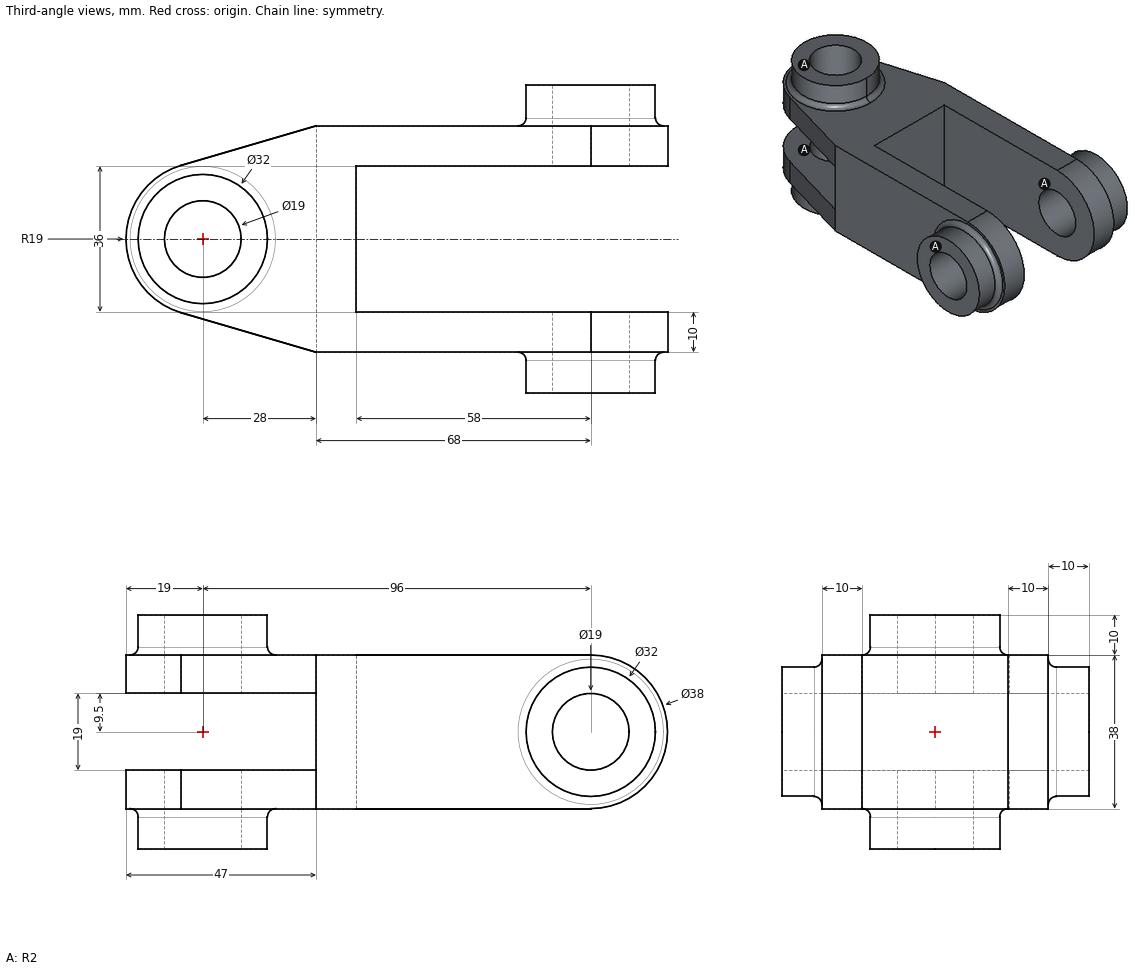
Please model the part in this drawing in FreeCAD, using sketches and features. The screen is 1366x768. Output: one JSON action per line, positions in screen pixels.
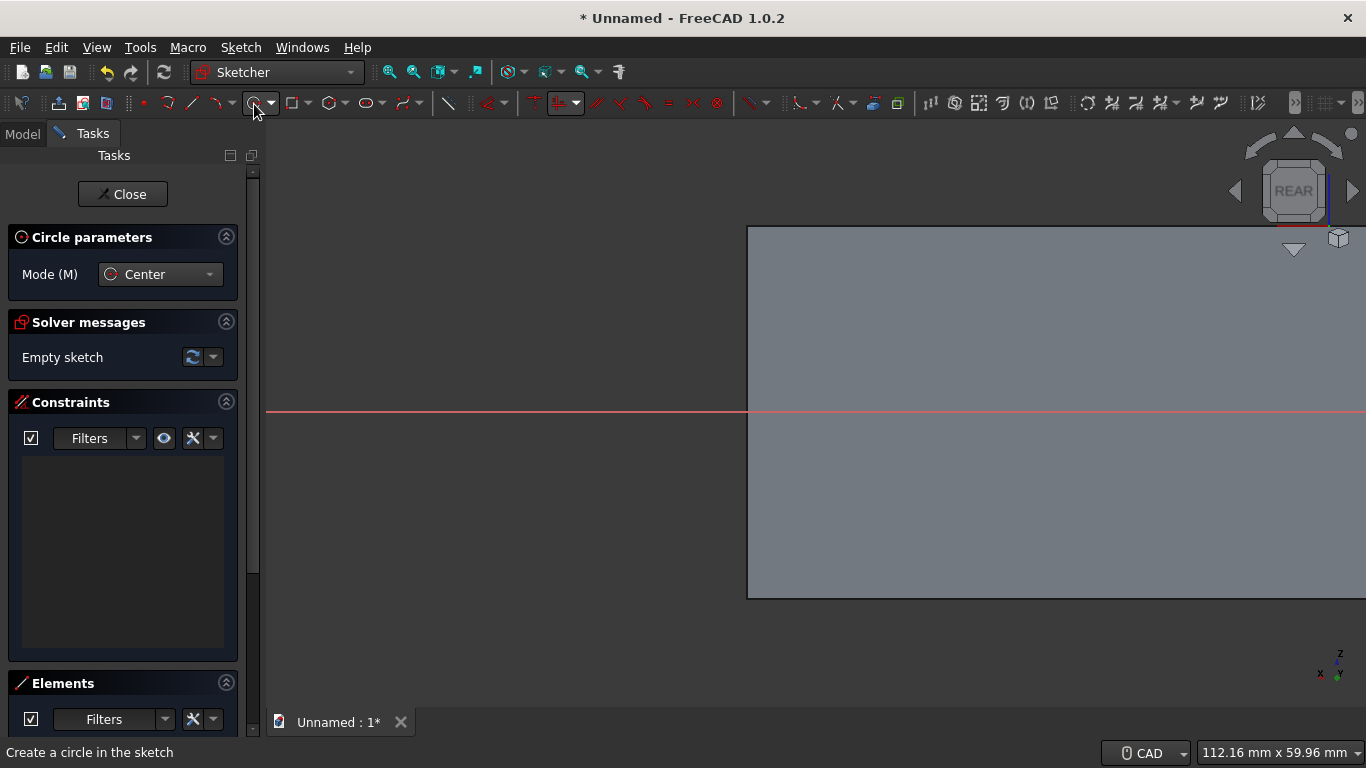
{"action": "left_click", "coordinate": [747, 412]}
{"action": "left_click", "coordinate": [879, 281]}
{"action": "key", "text": "Escape"}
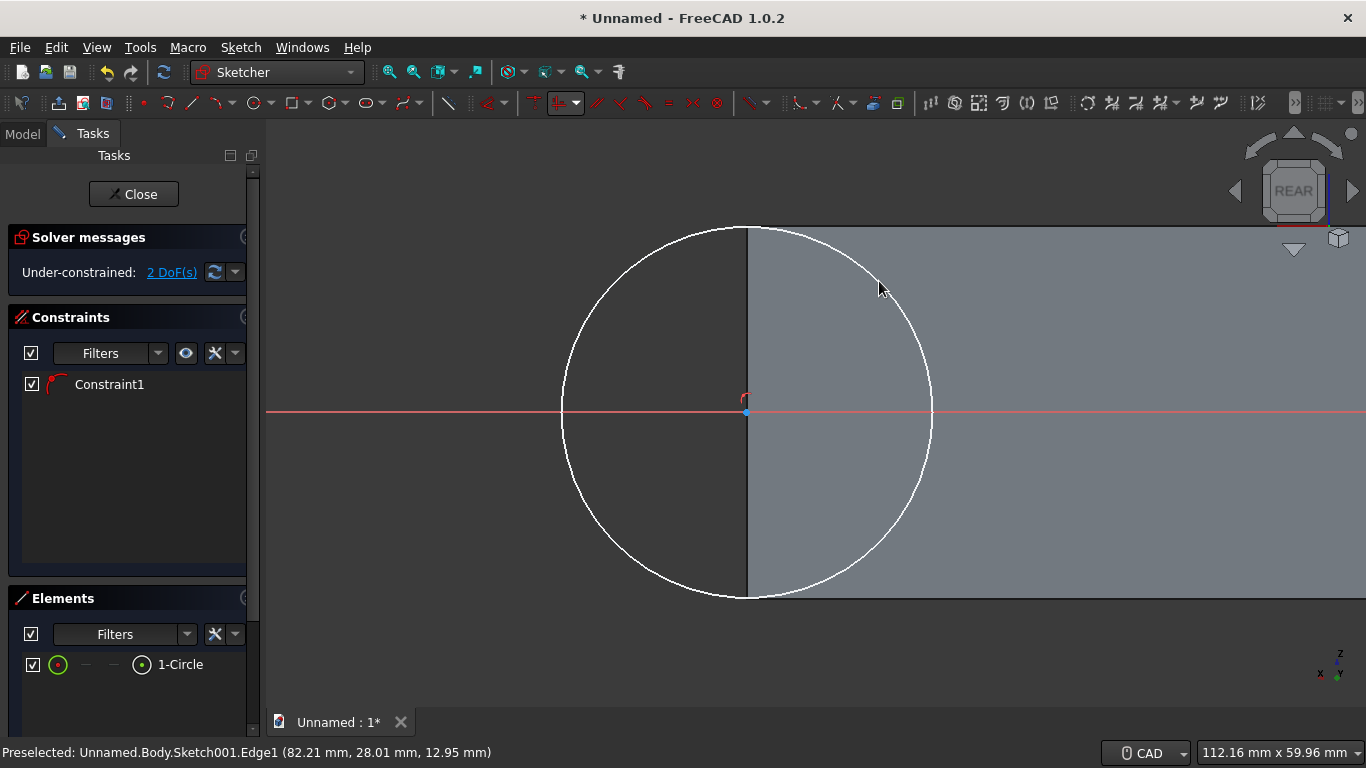
{"action": "key", "text": "d"}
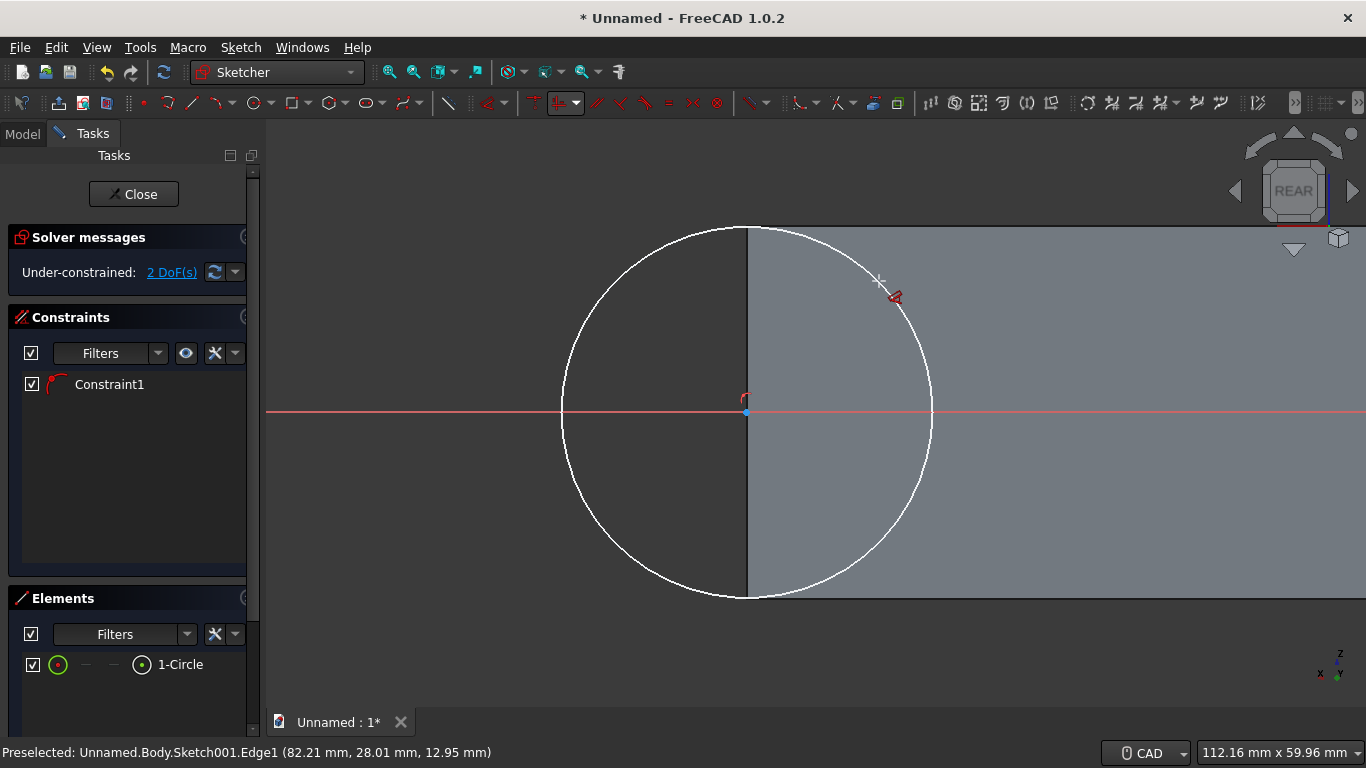
{"action": "left_click", "coordinate": [878, 281]}
{"action": "left_click", "coordinate": [901, 258]}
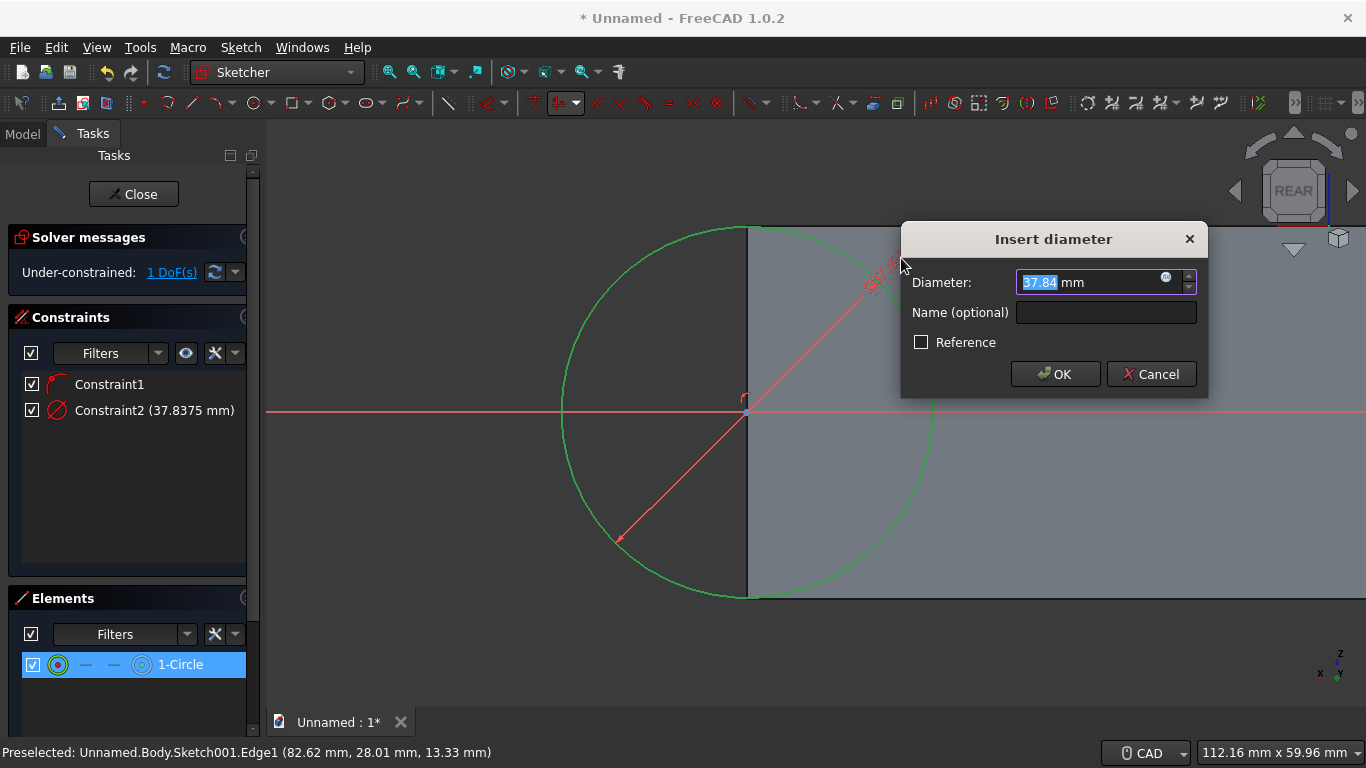
{"action": "type", "text": "38"}
{"action": "key", "text": "Return"}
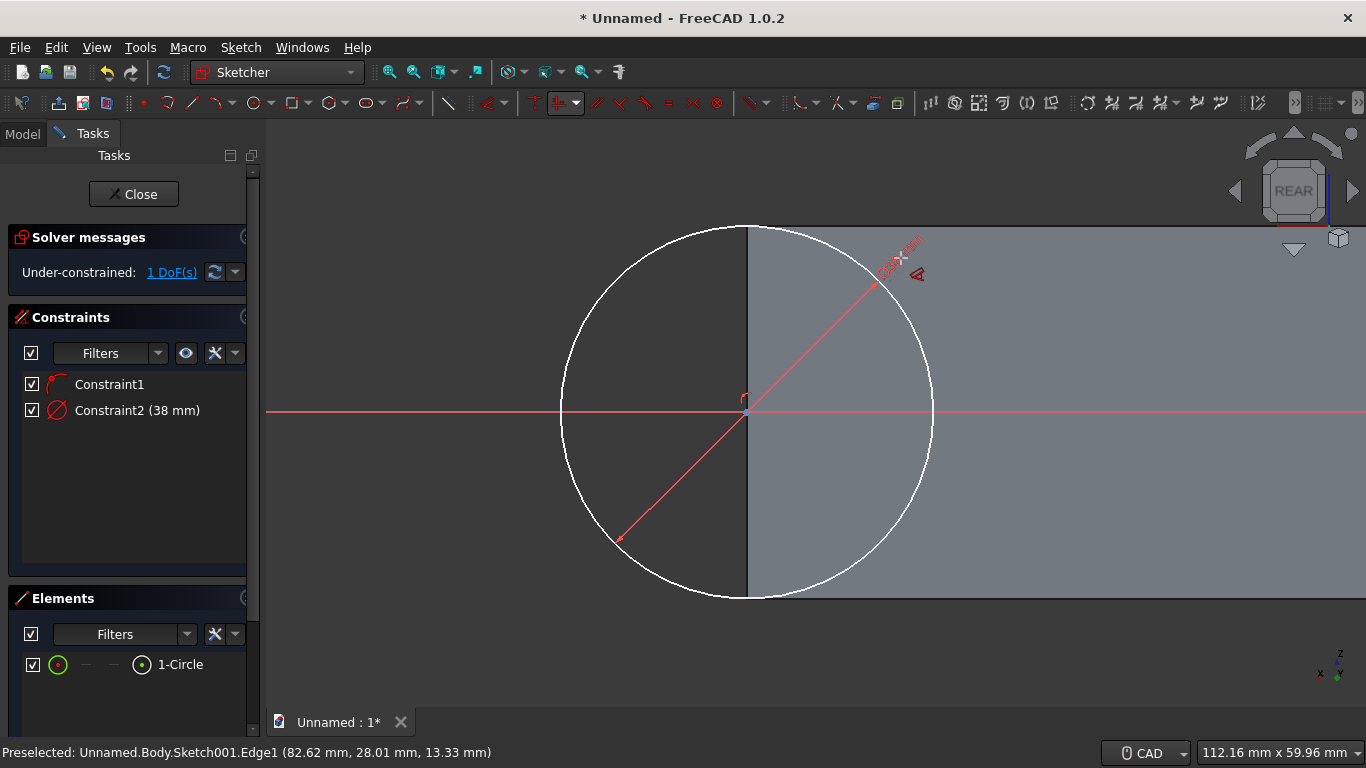
{"action": "left_click", "coordinate": [747, 412]}
{"action": "left_click", "coordinate": [974, 446]}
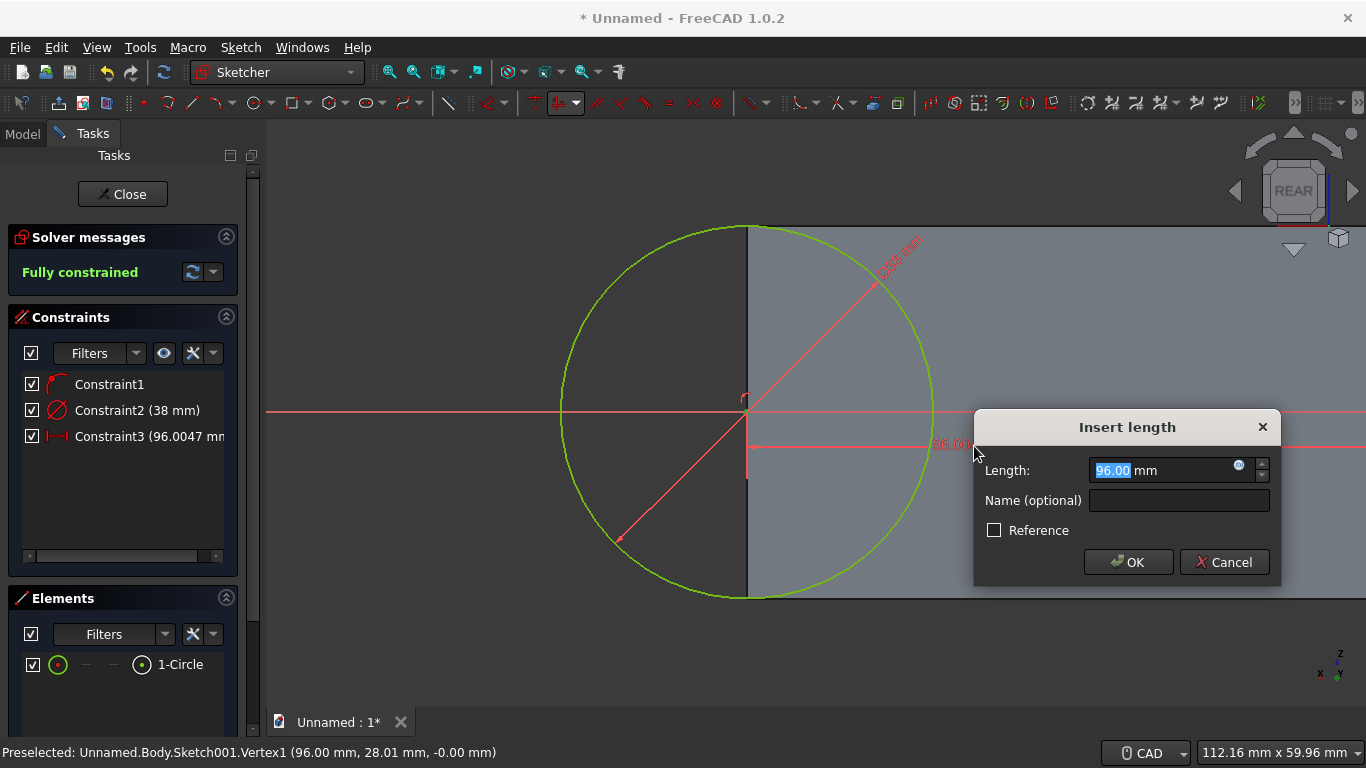
{"action": "type", "text": "96"}
{"action": "key", "text": "Return"}
{"action": "key", "text": "Escape"}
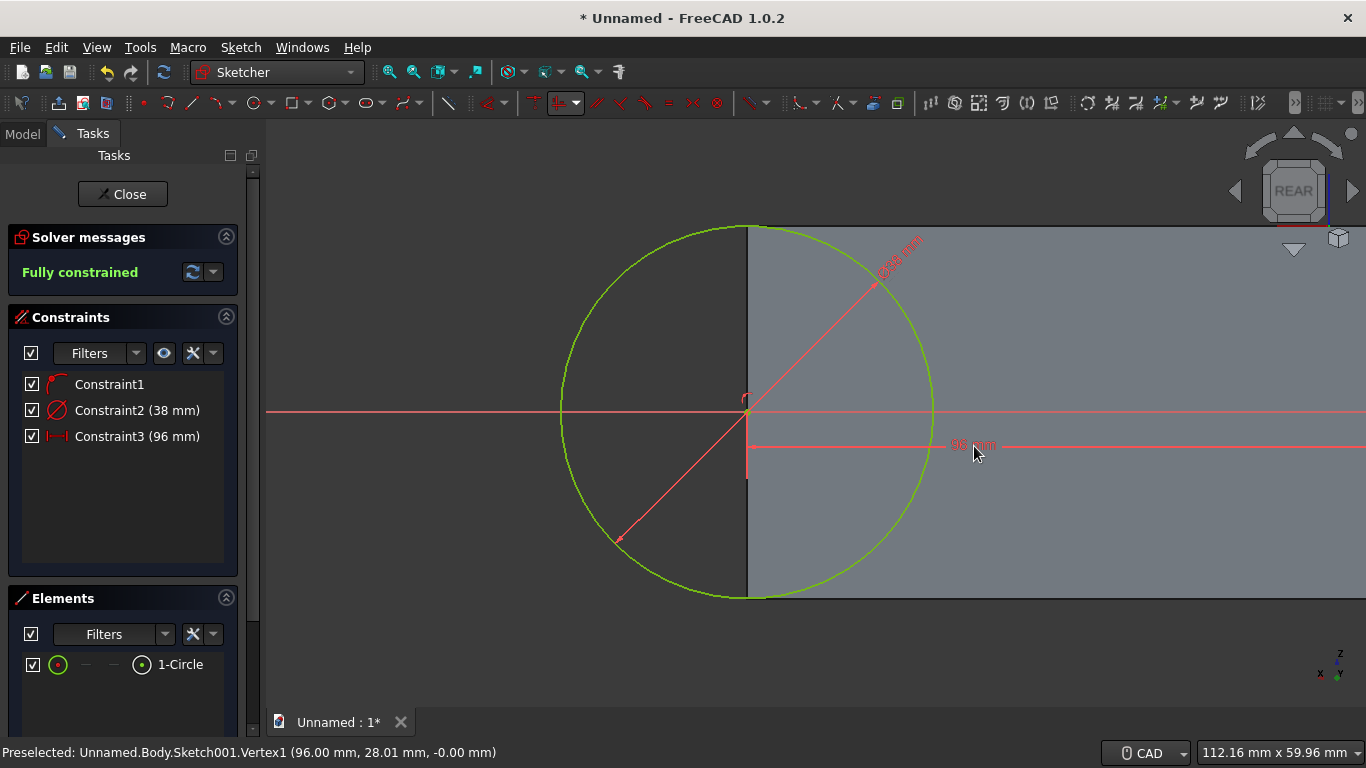
{"action": "left_click", "coordinate": [123, 194]}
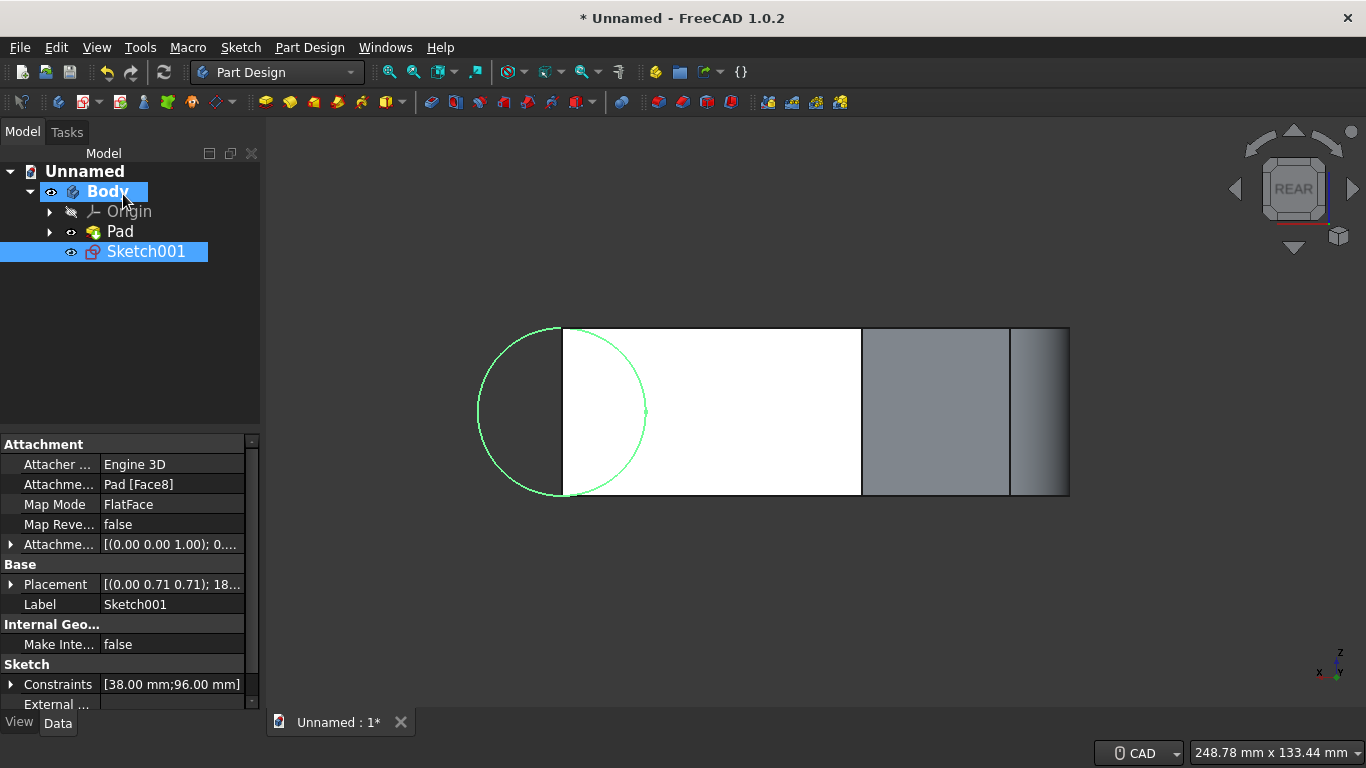
{"action": "left_click", "coordinate": [266, 102]}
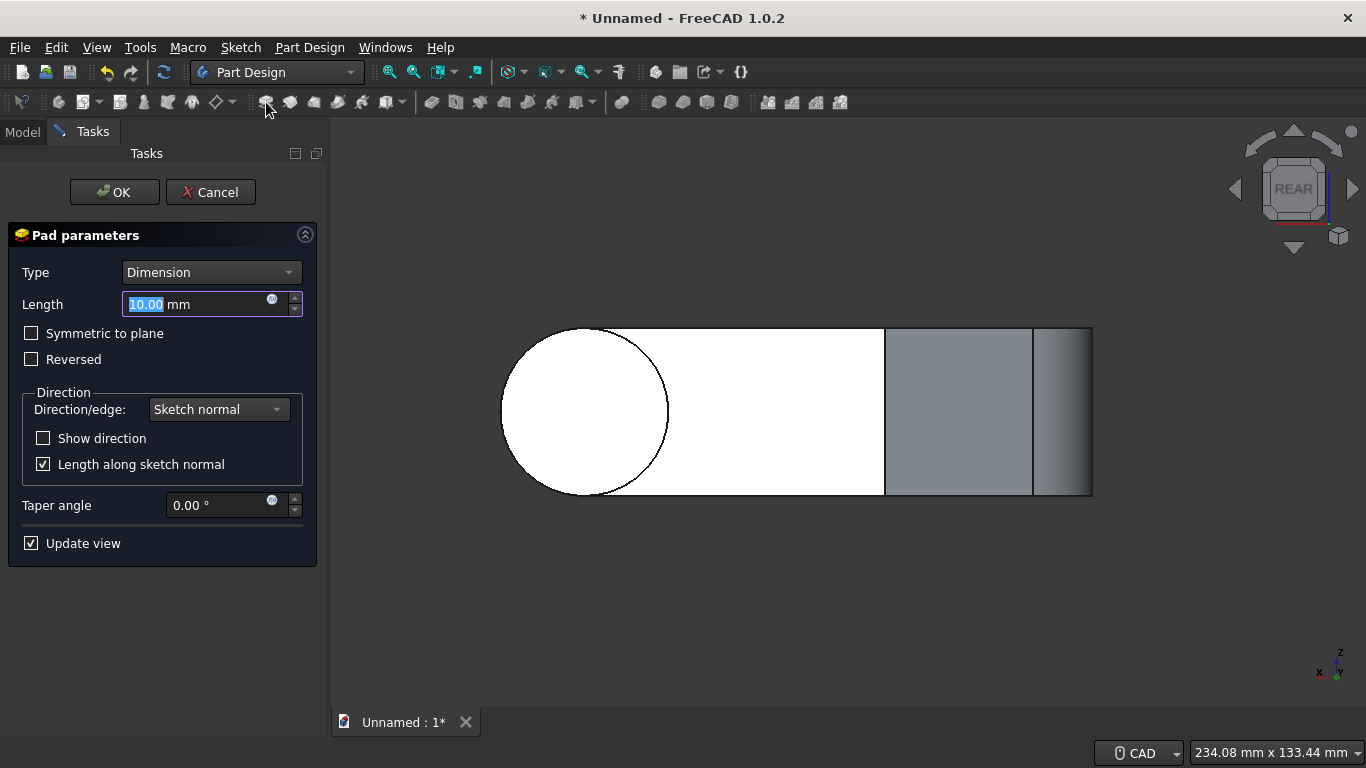
{"action": "type", "text": "10"}
{"action": "key", "text": "Tab"}